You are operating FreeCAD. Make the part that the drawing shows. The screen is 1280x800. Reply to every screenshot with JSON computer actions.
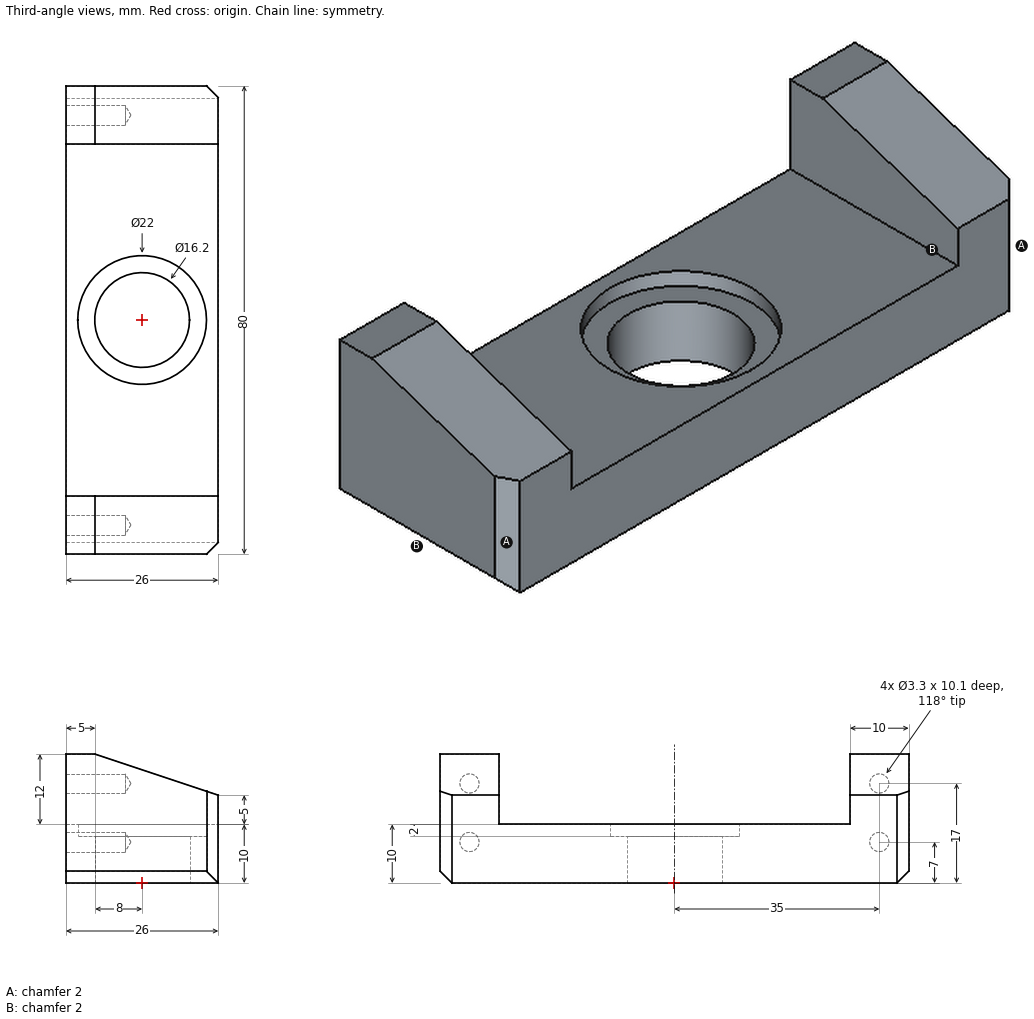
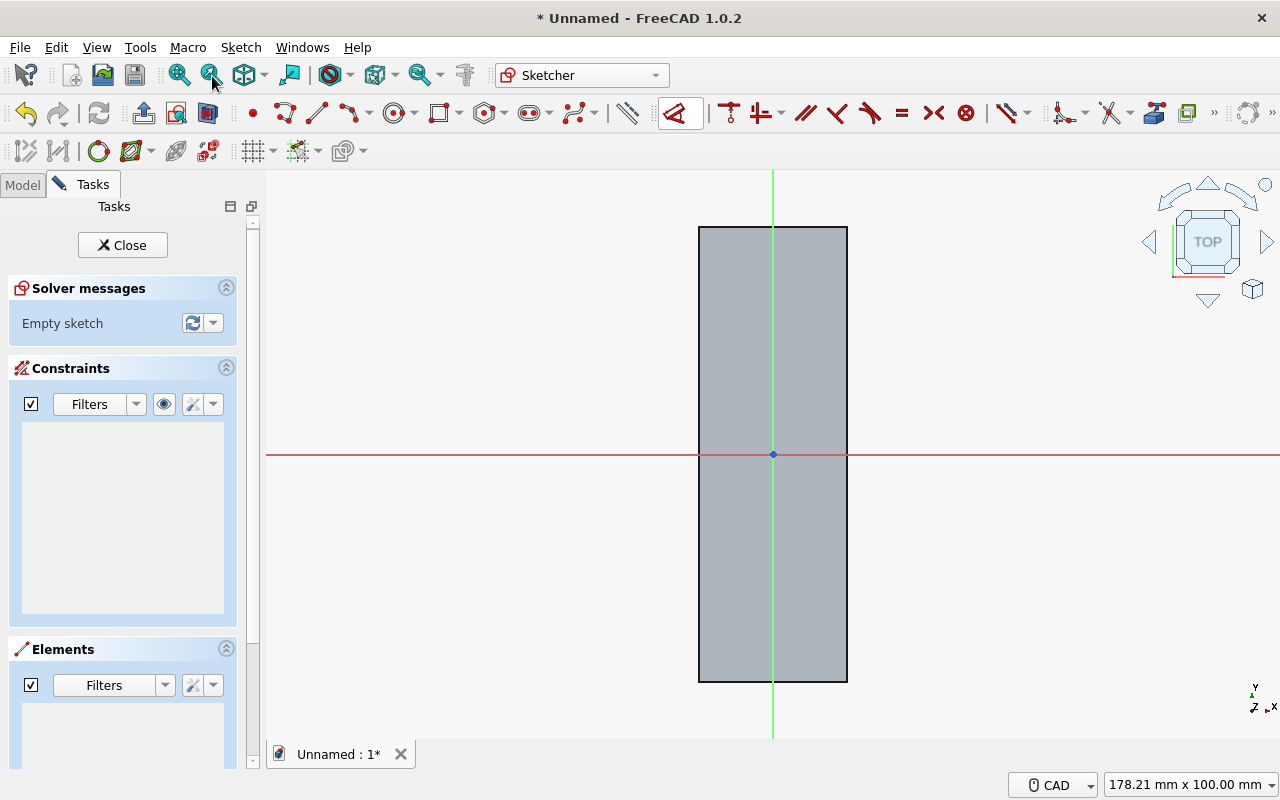
{"action": "scroll", "coordinate": [795, 454], "scroll_direction": "up", "scroll_amount": 7}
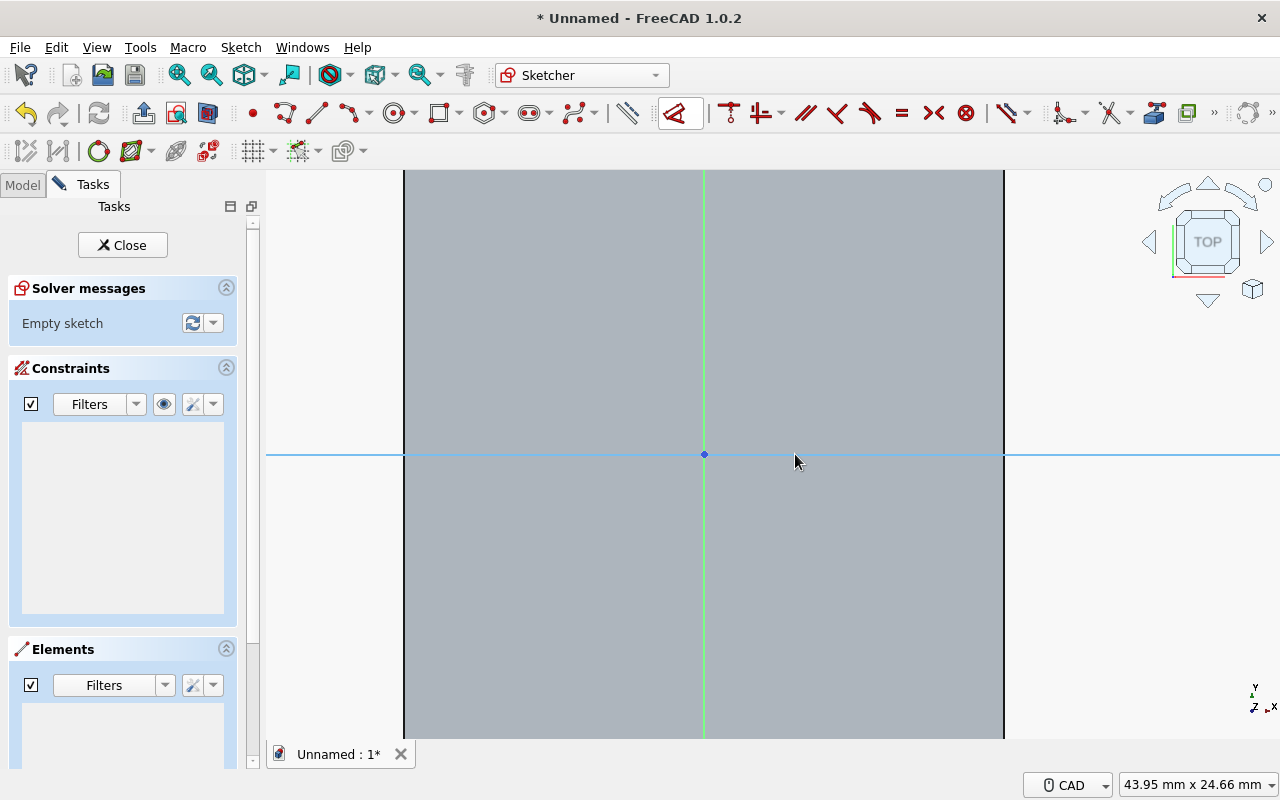
{"action": "left_click", "coordinate": [394, 114]}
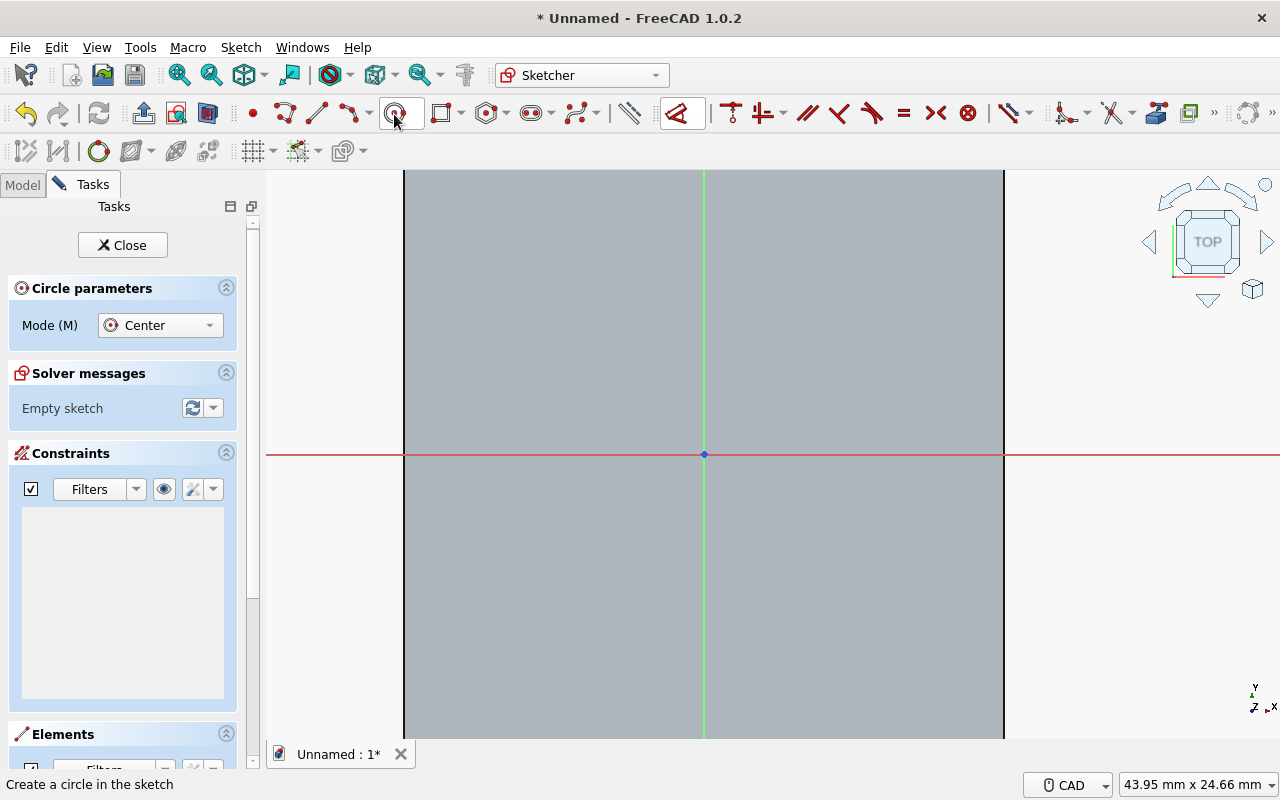
{"action": "left_click", "coordinate": [704, 454]}
{"action": "left_click", "coordinate": [836, 322]}
{"action": "key", "text": "Escape"}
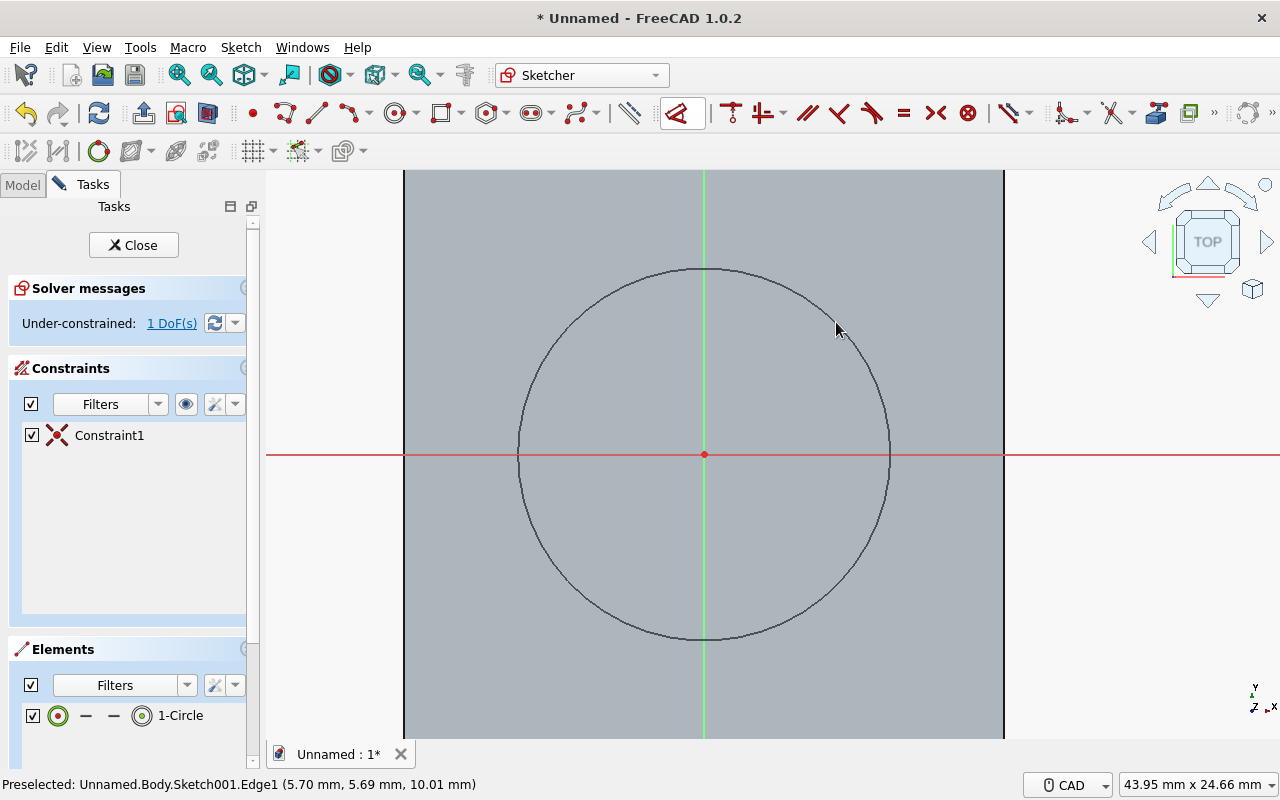
{"action": "left_click", "coordinate": [835, 322]}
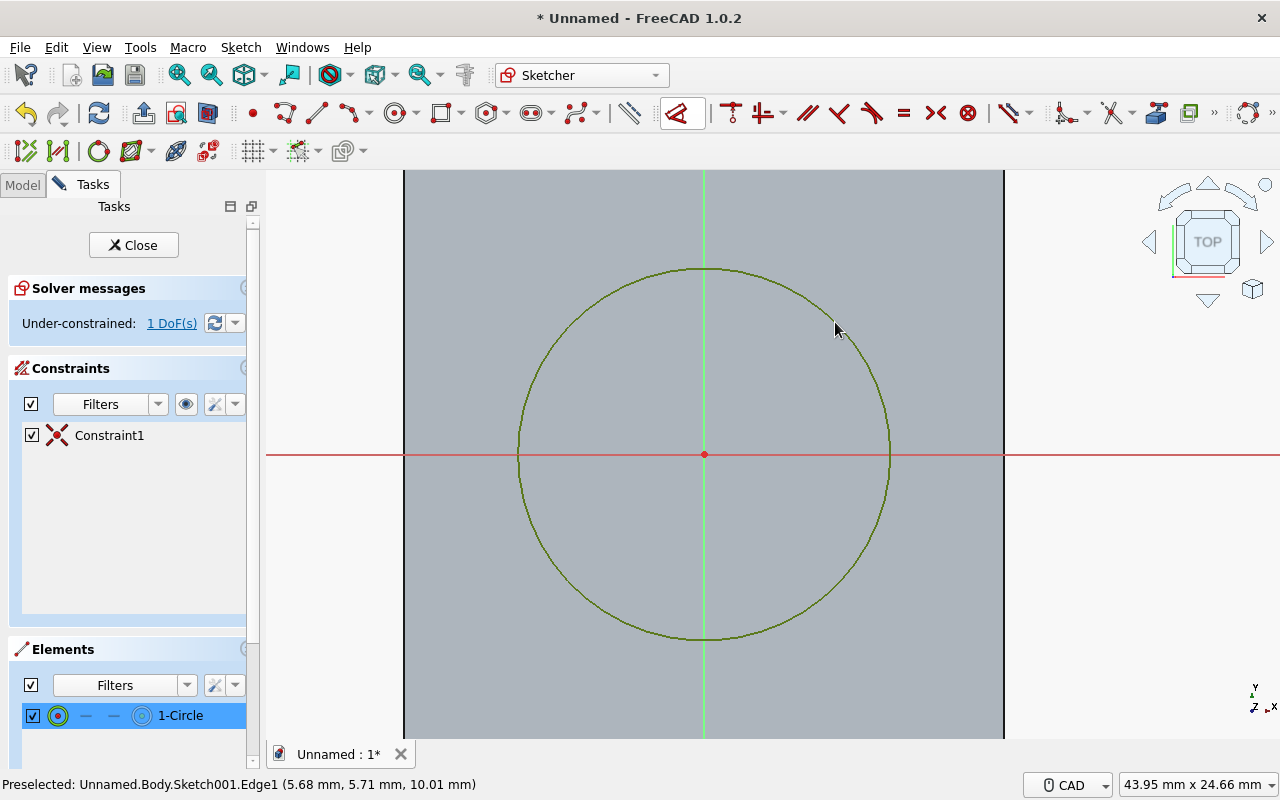
{"action": "key", "text": "k o"}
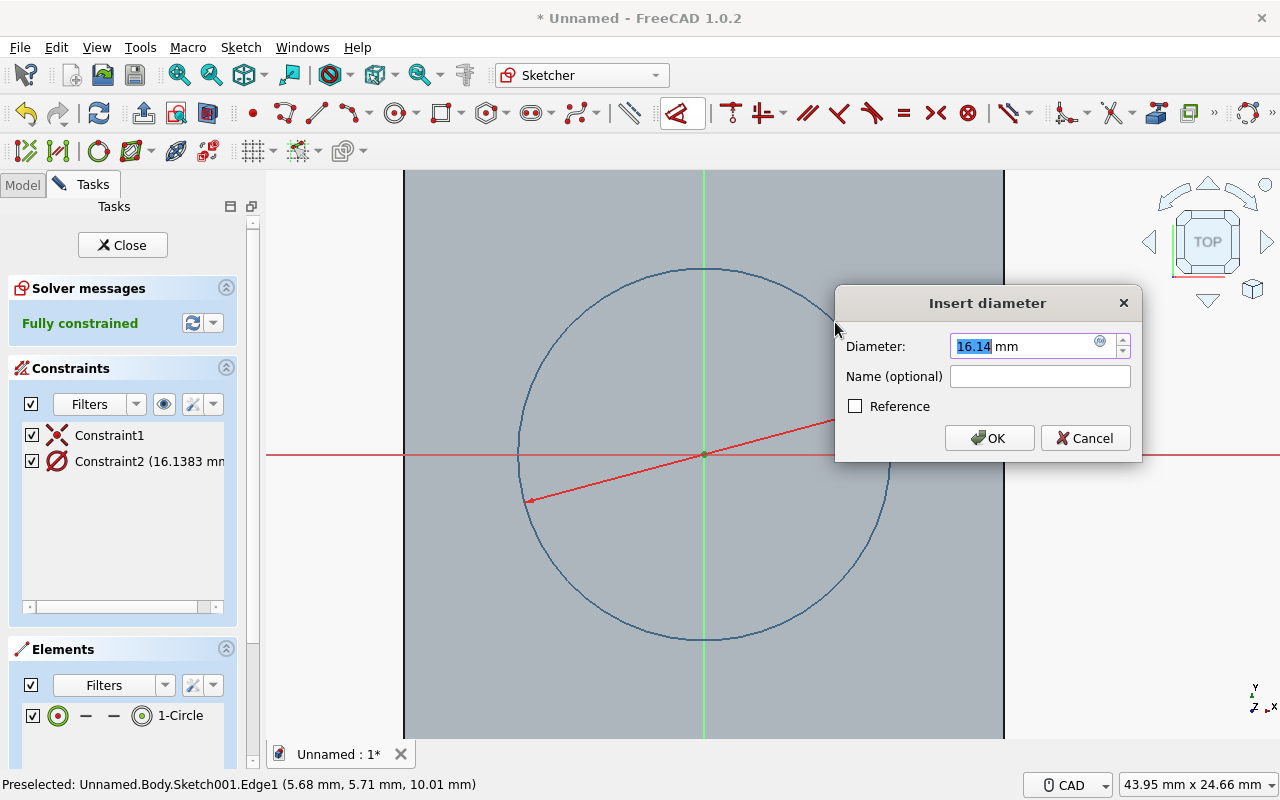
{"action": "type", "text": "16.2"}
{"action": "key", "text": "Return"}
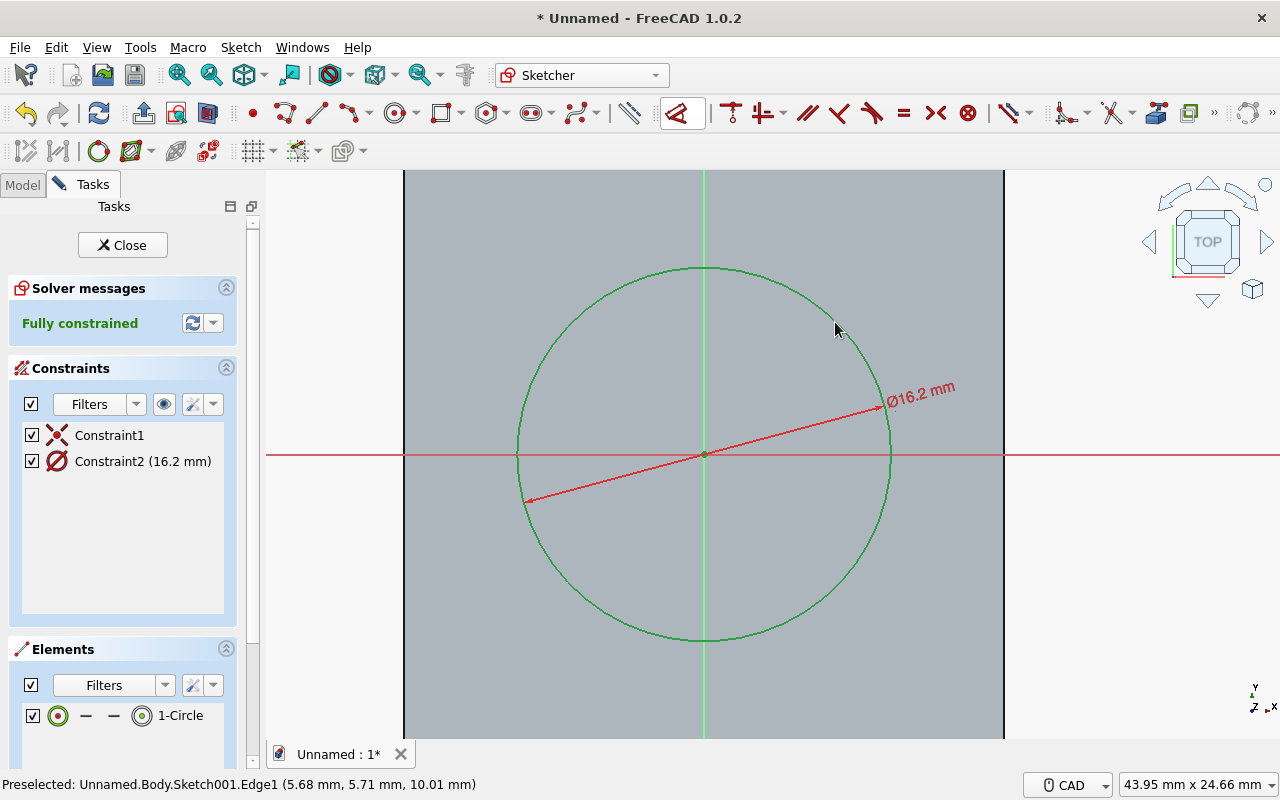
{"action": "left_click", "coordinate": [123, 245]}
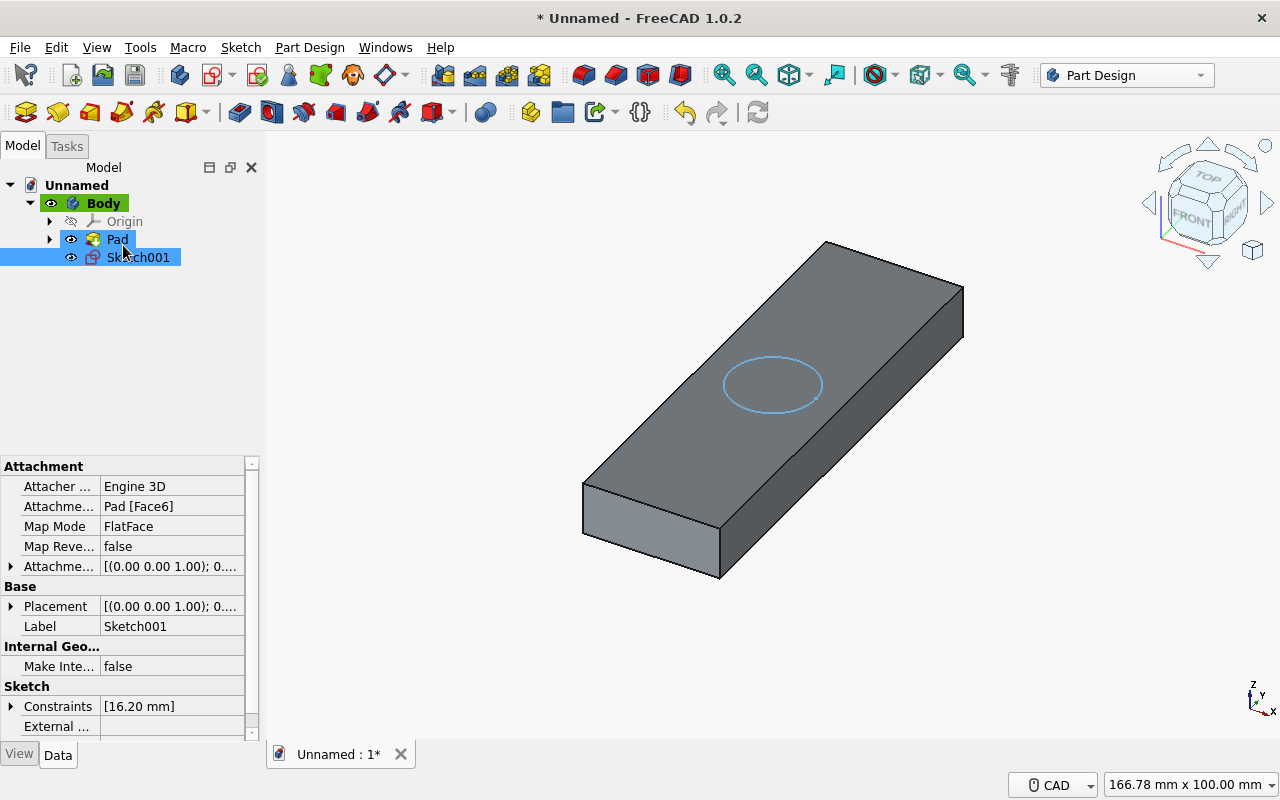
{"action": "left_click", "coordinate": [240, 112]}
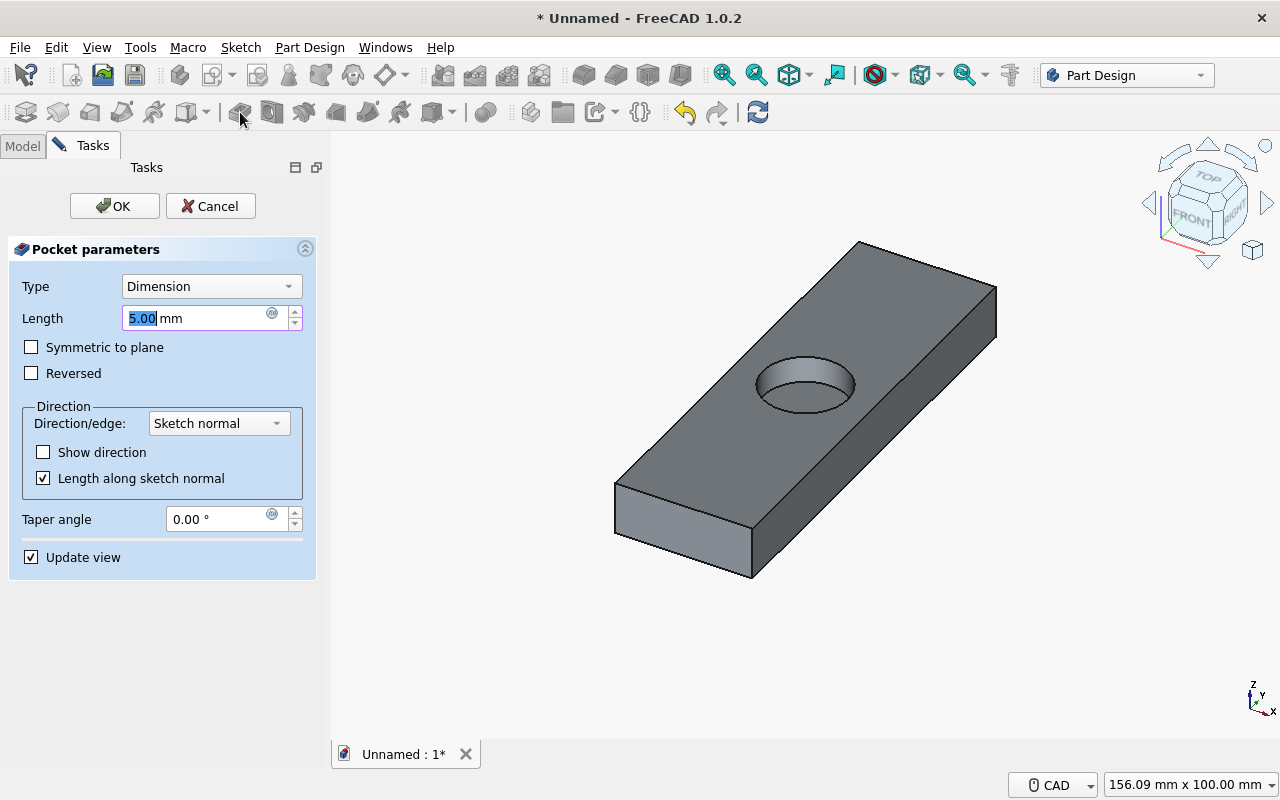
{"action": "left_click", "coordinate": [212, 286]}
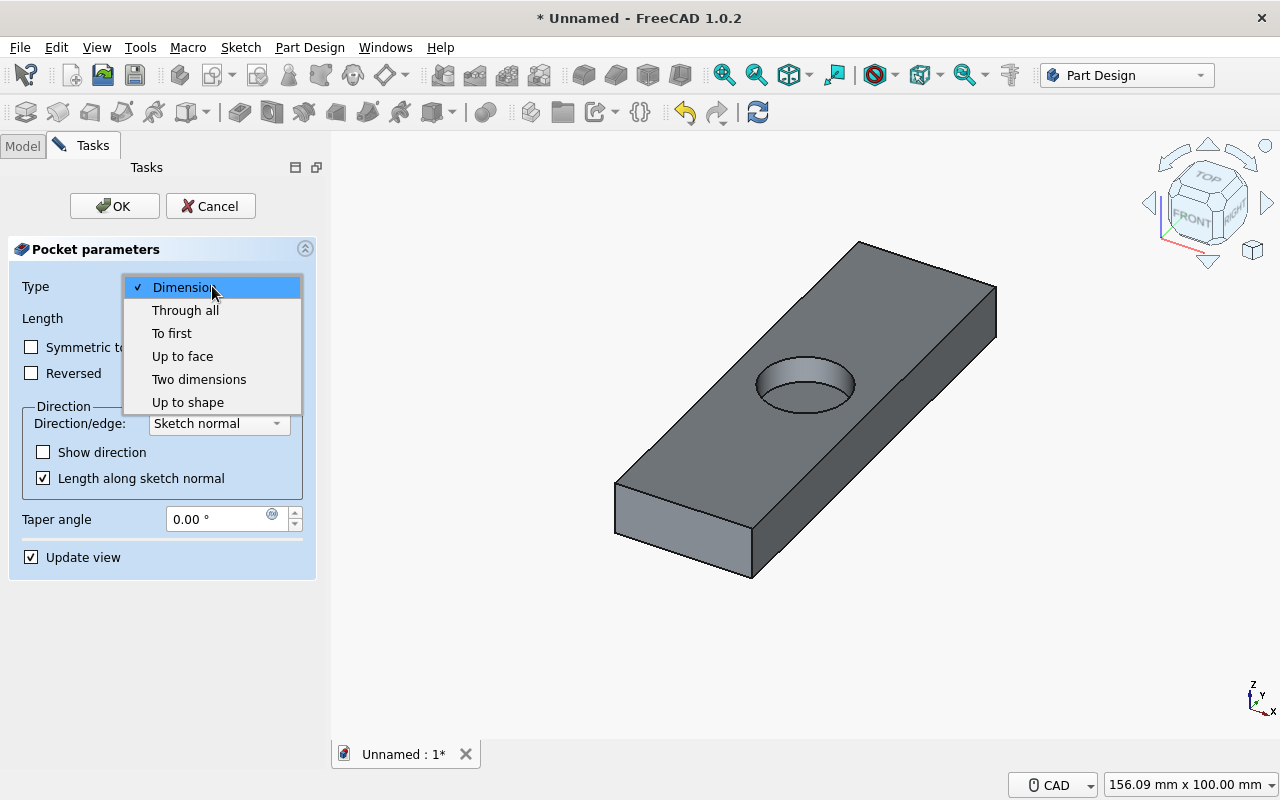
{"action": "left_click", "coordinate": [212, 310]}